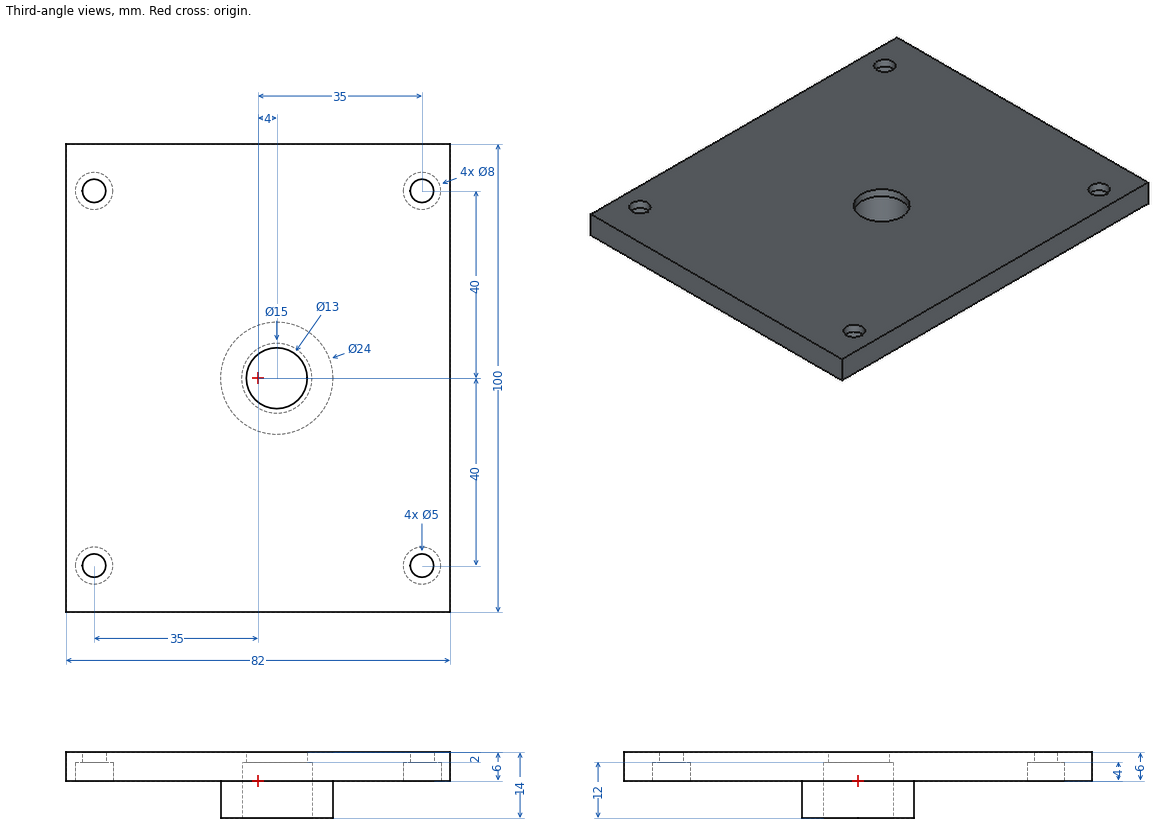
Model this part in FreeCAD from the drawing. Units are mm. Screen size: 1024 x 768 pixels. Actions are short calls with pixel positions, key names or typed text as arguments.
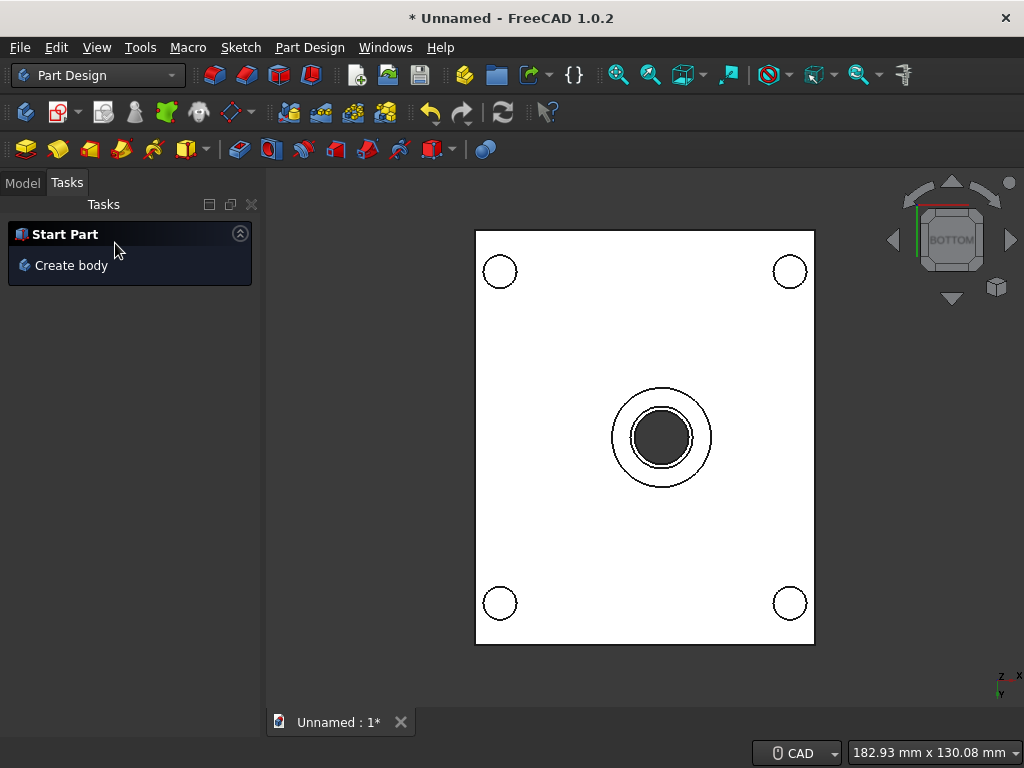
click(596, 555)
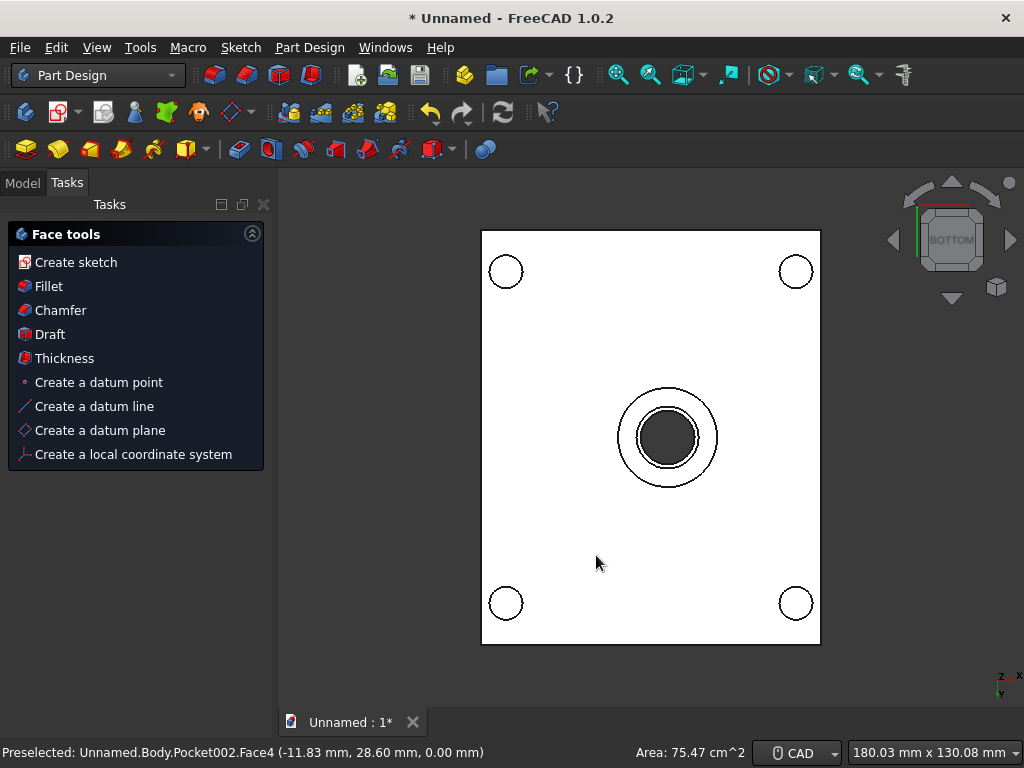
click(58, 112)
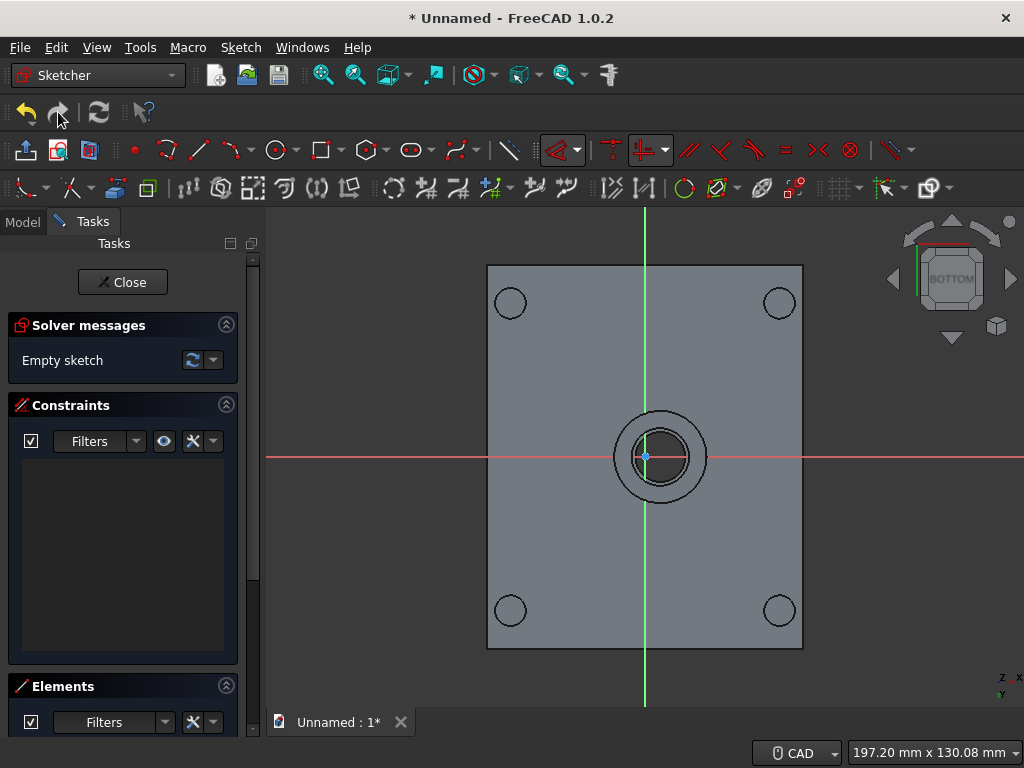
click(276, 150)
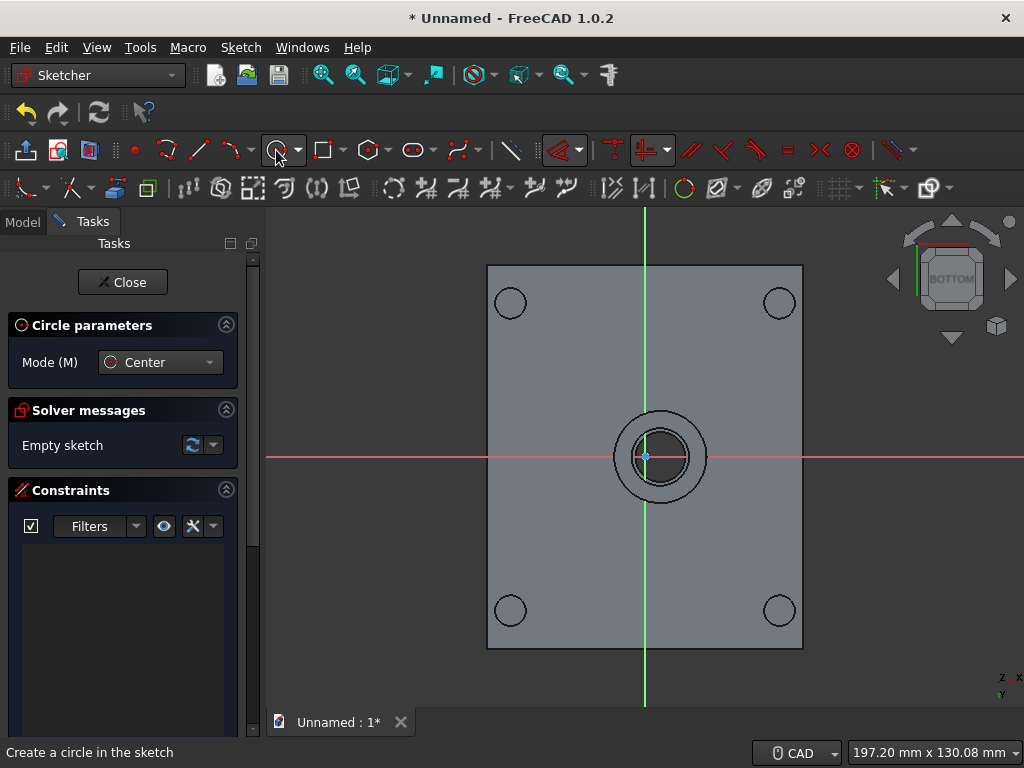
scroll(780, 303, up, 5)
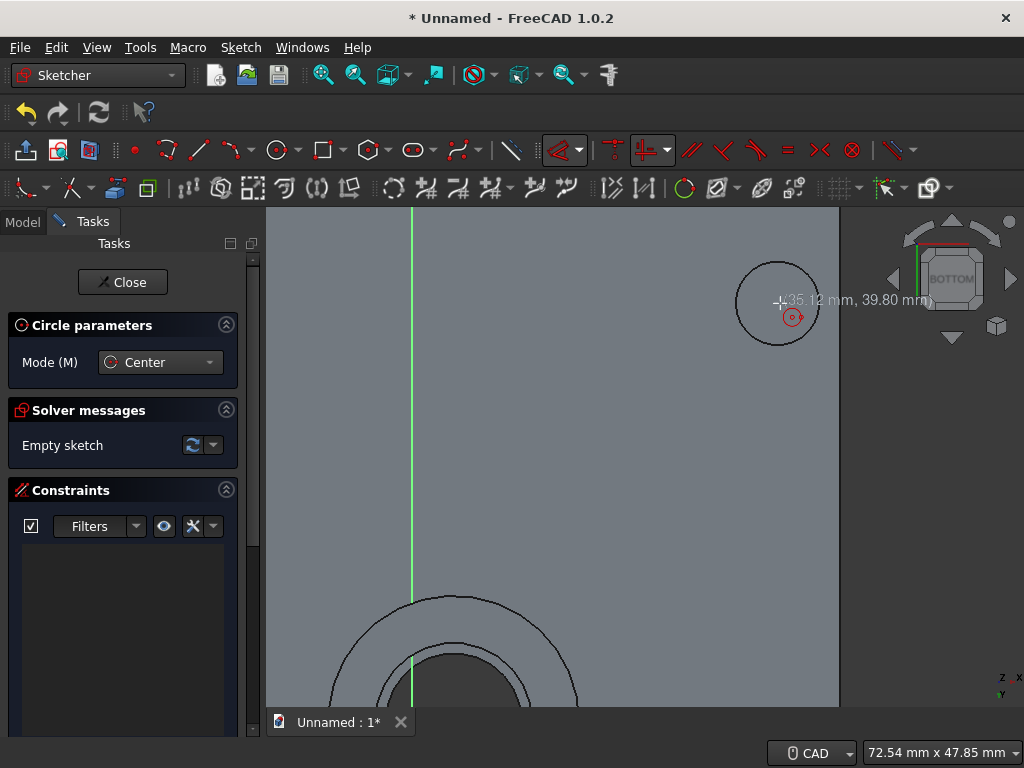
click(778, 303)
move(796, 285)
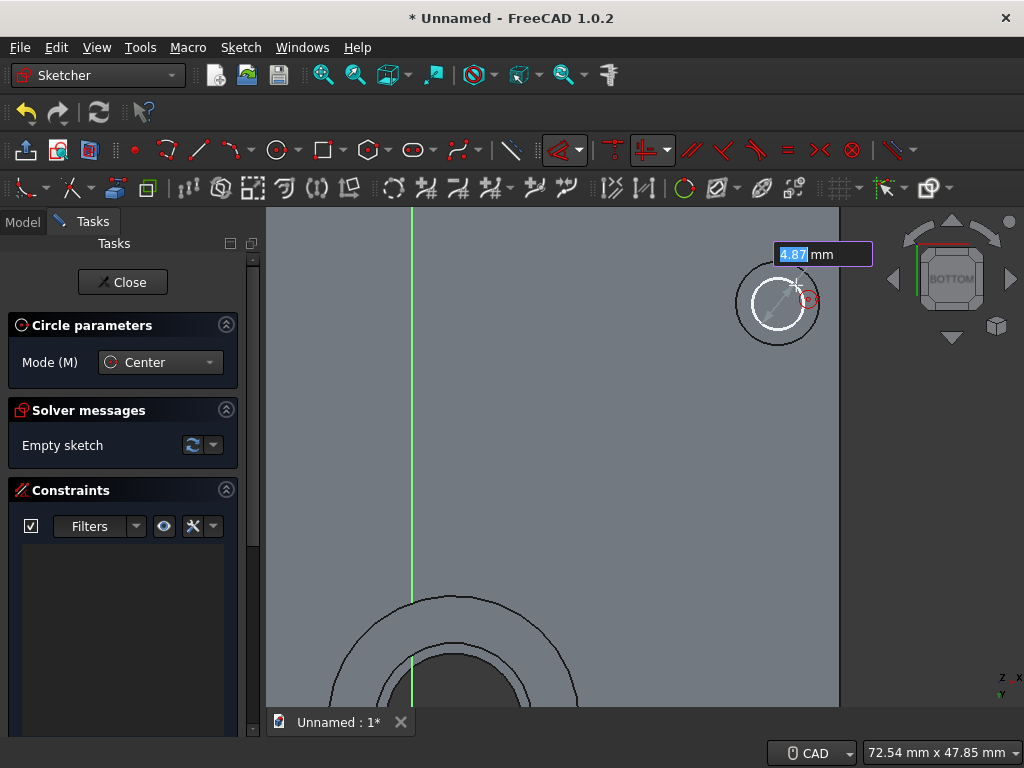
text(5)
key(Return)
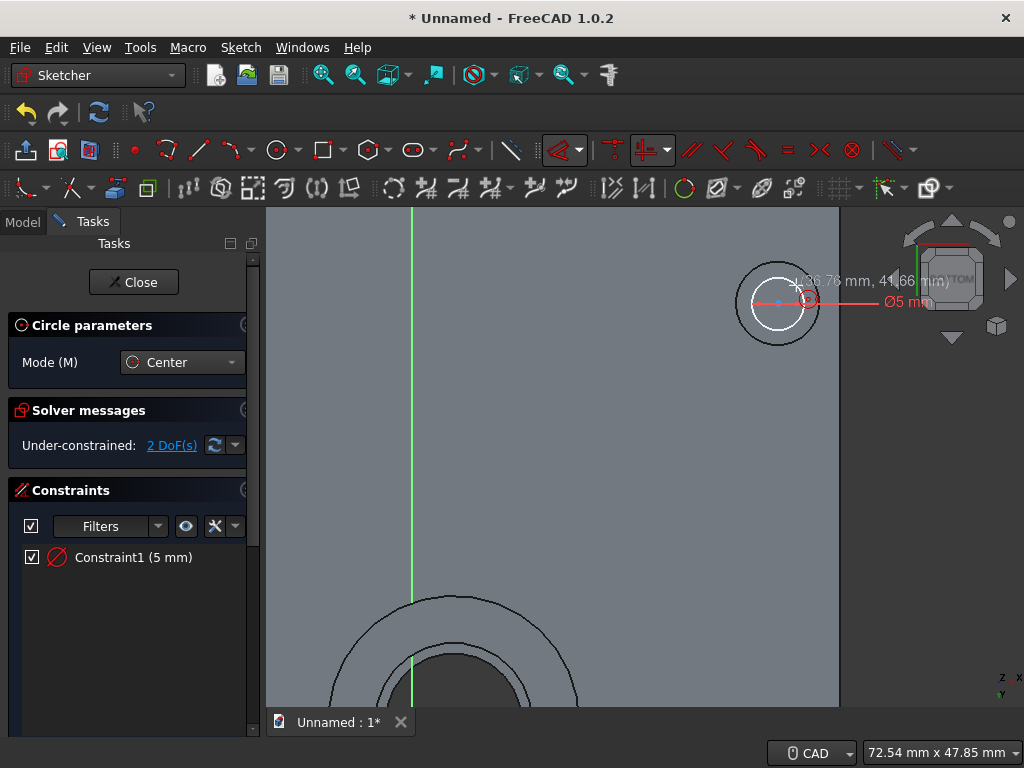
scroll(672, 303, down, 5)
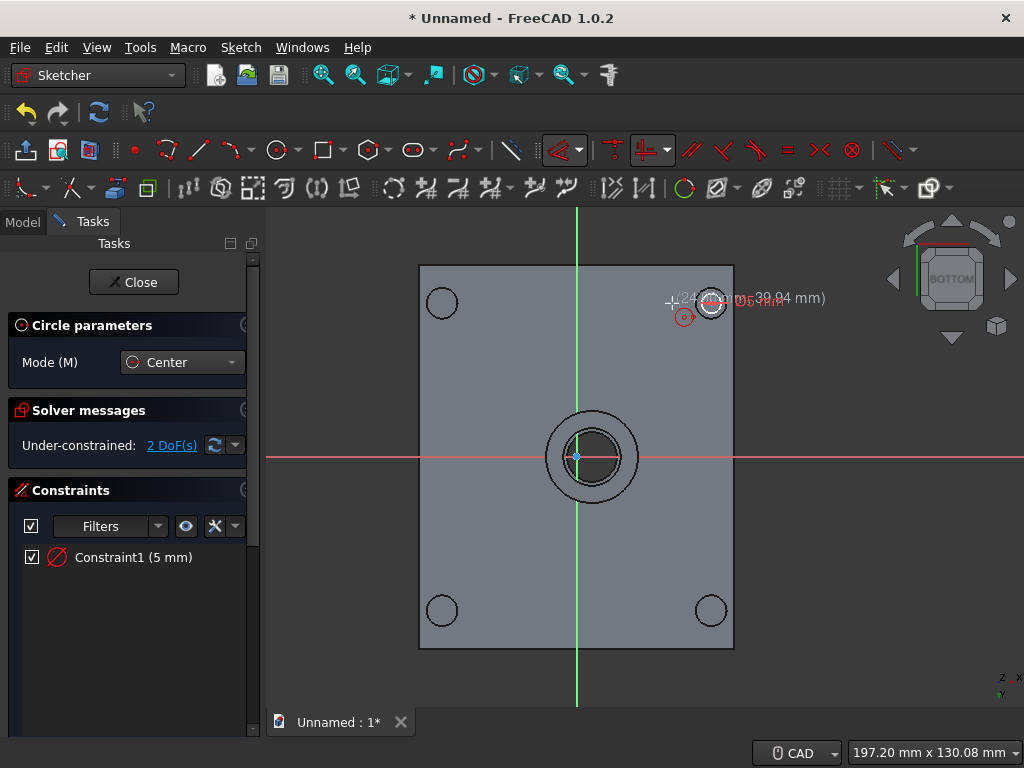
scroll(711, 611, up, 5)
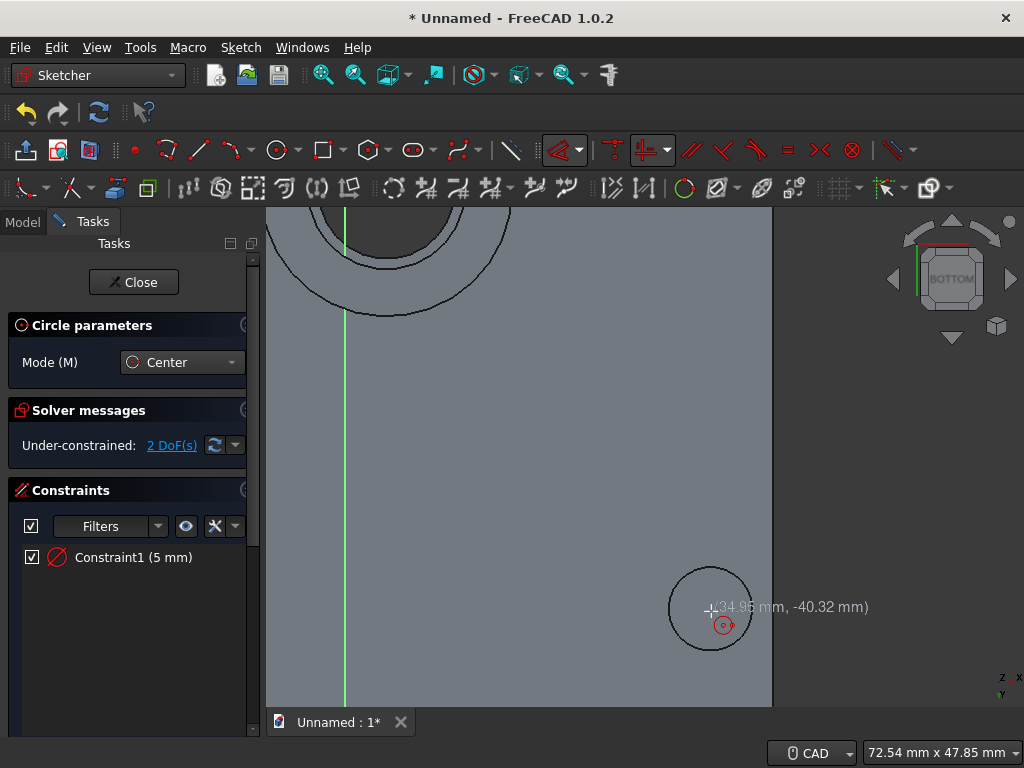
click(710, 609)
move(729, 590)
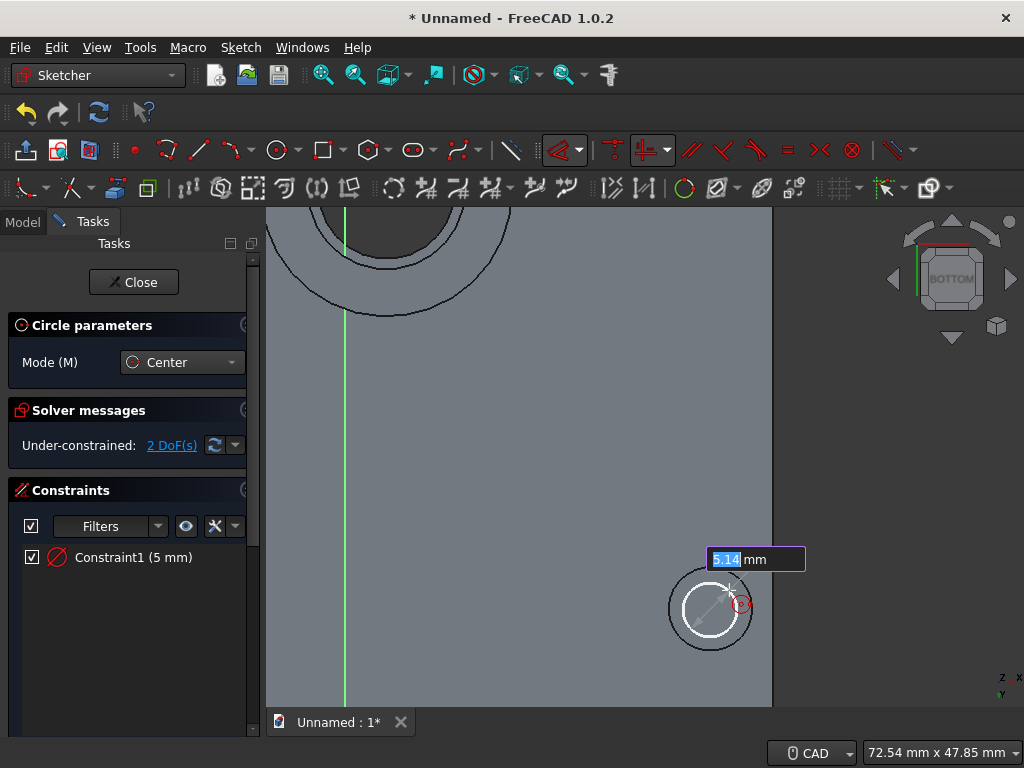
text(5)
key(Return)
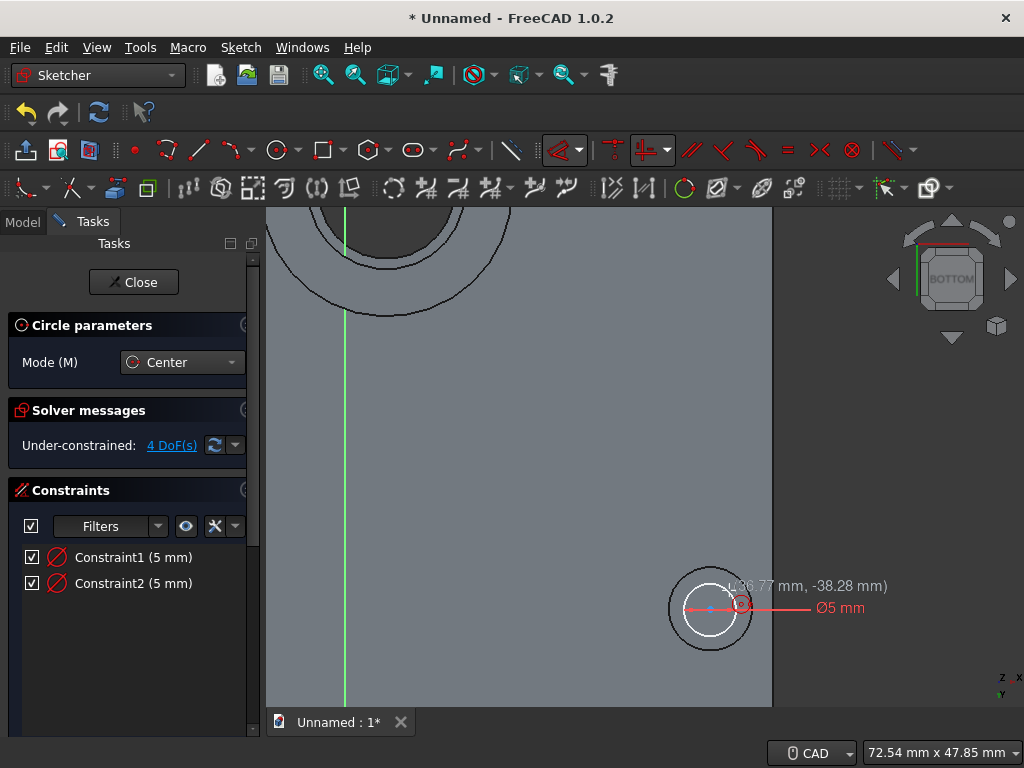
scroll(711, 612, down, 5)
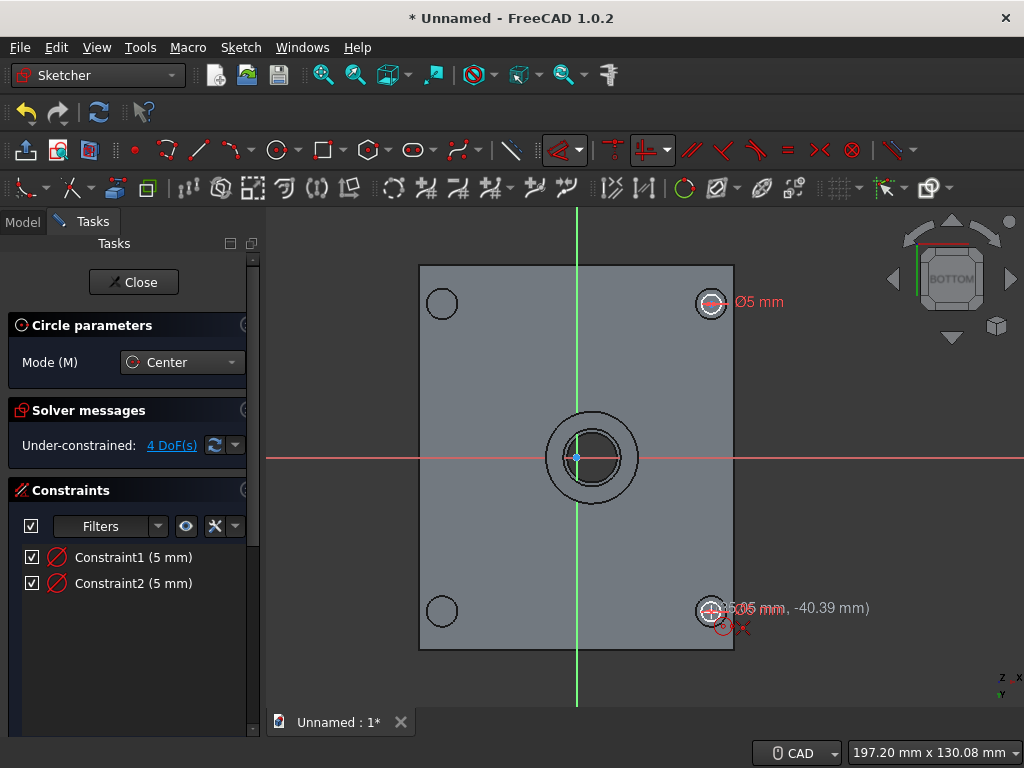
scroll(442, 304, up, 5)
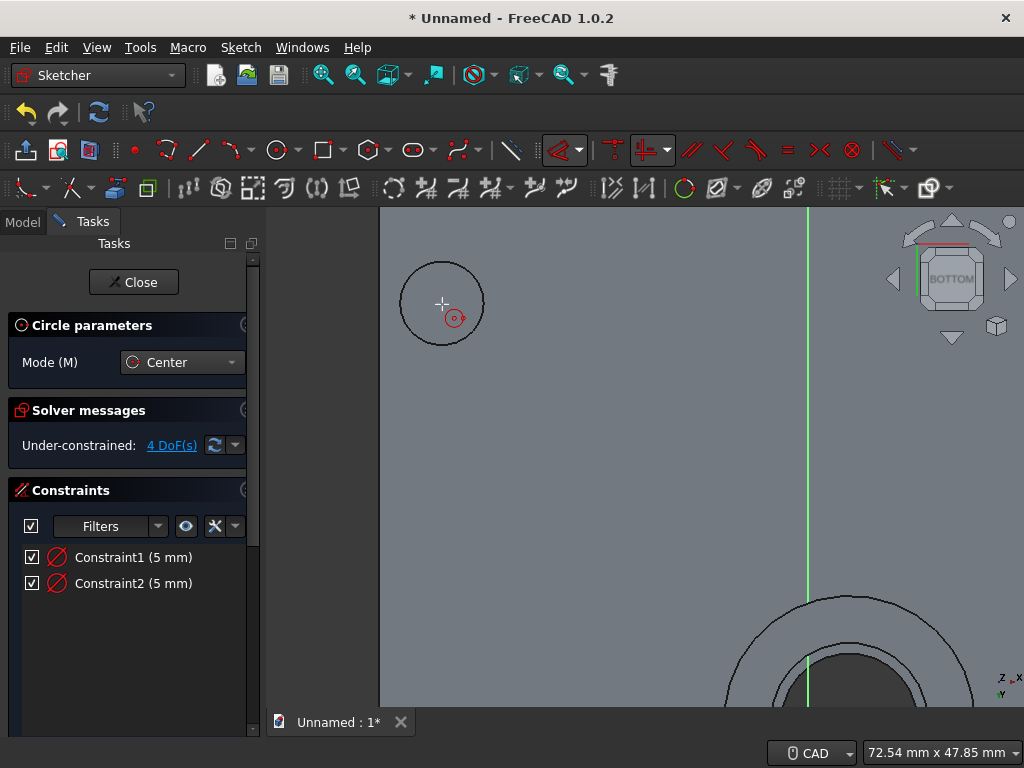
click(442, 303)
move(460, 285)